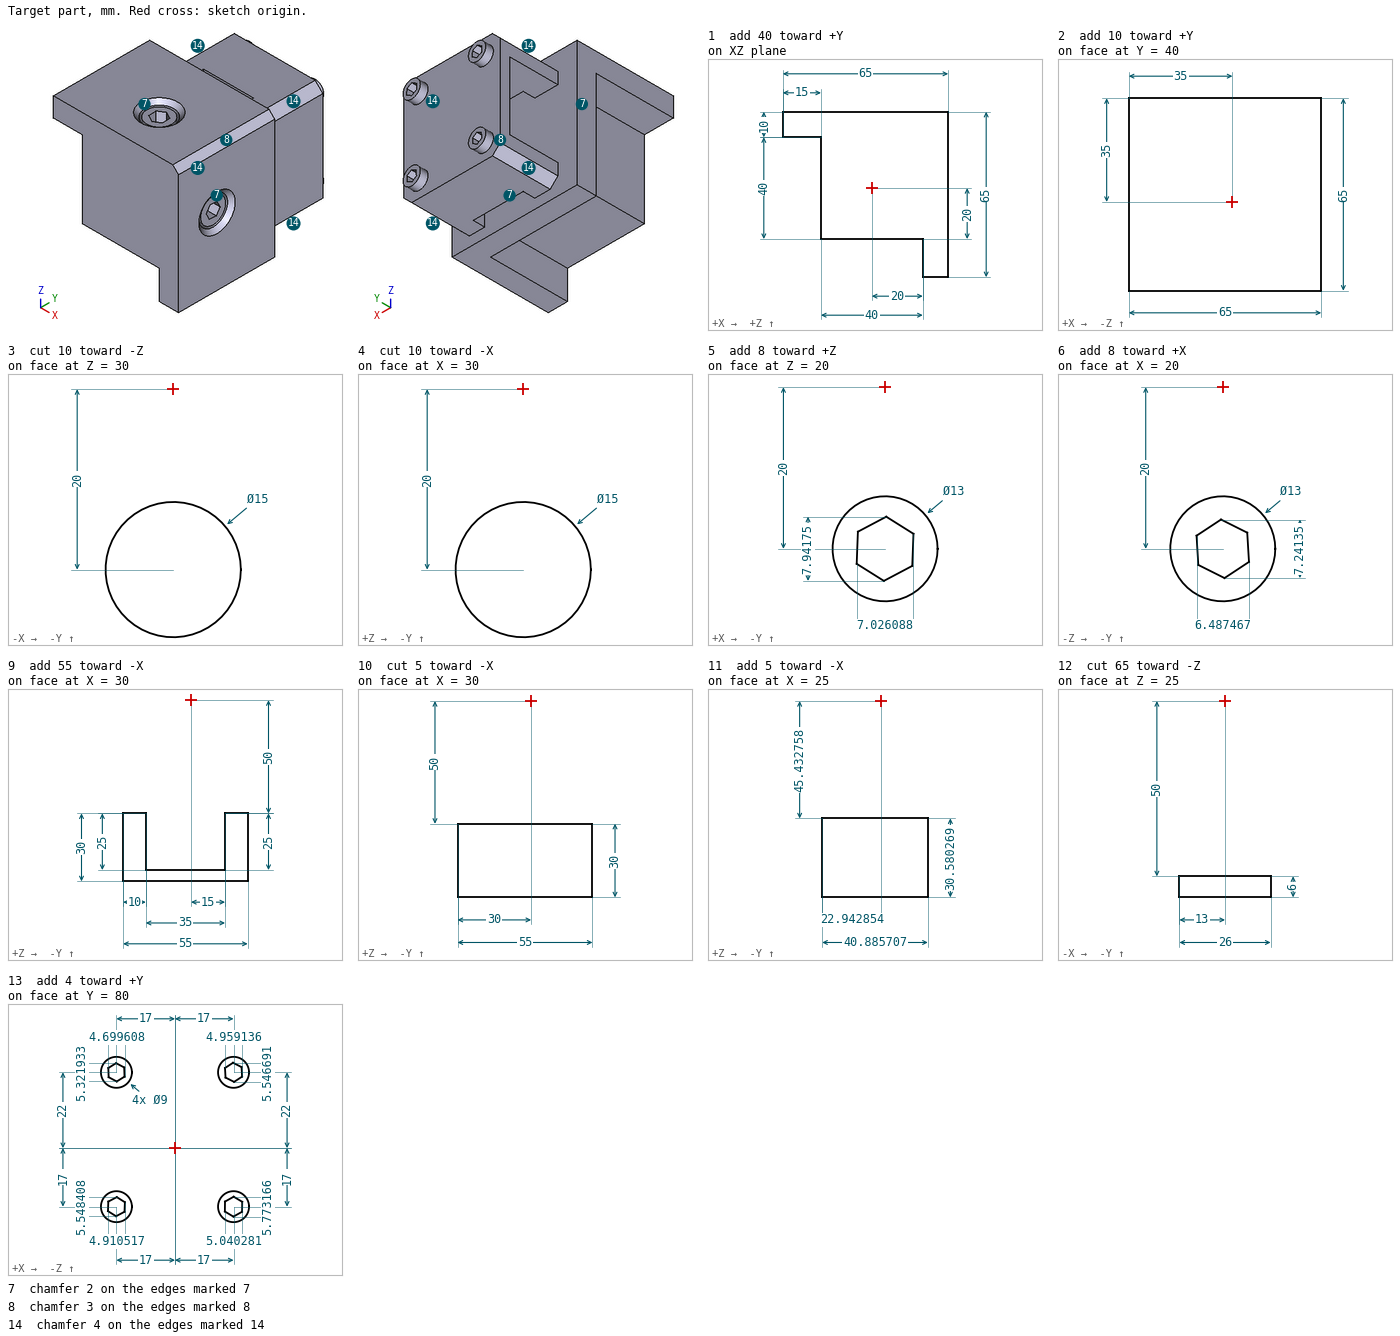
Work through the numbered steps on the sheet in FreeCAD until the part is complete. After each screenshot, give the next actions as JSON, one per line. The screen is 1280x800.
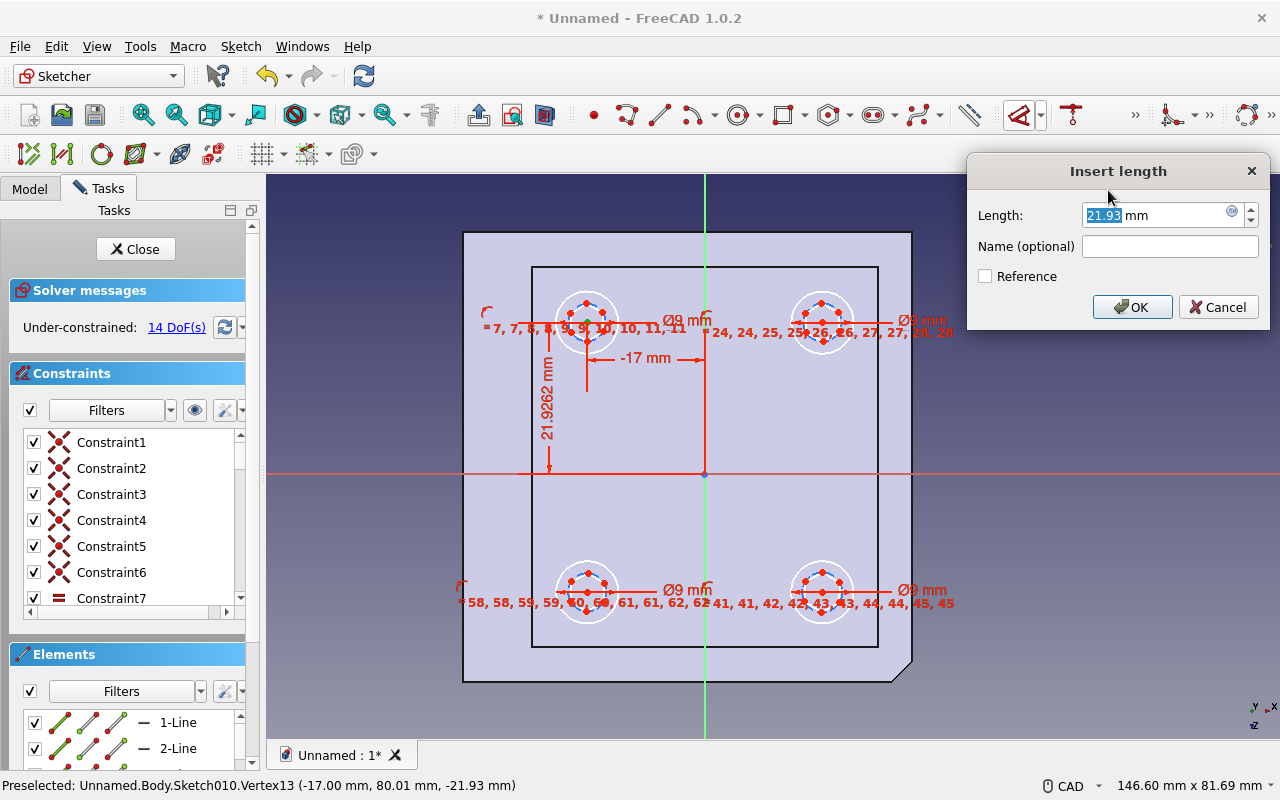
{"action": "type", "text": "22"}
{"action": "key", "text": "Return"}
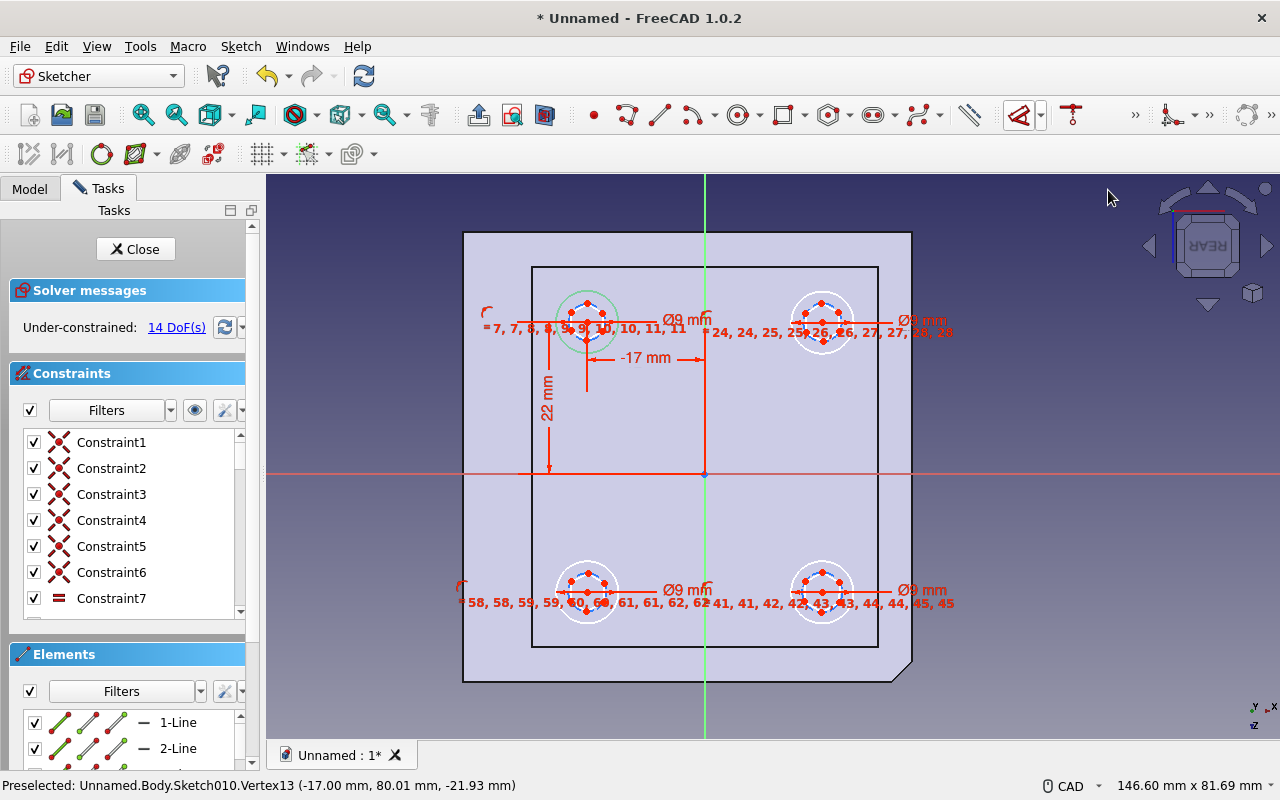
{"action": "left_click", "coordinate": [822, 323]}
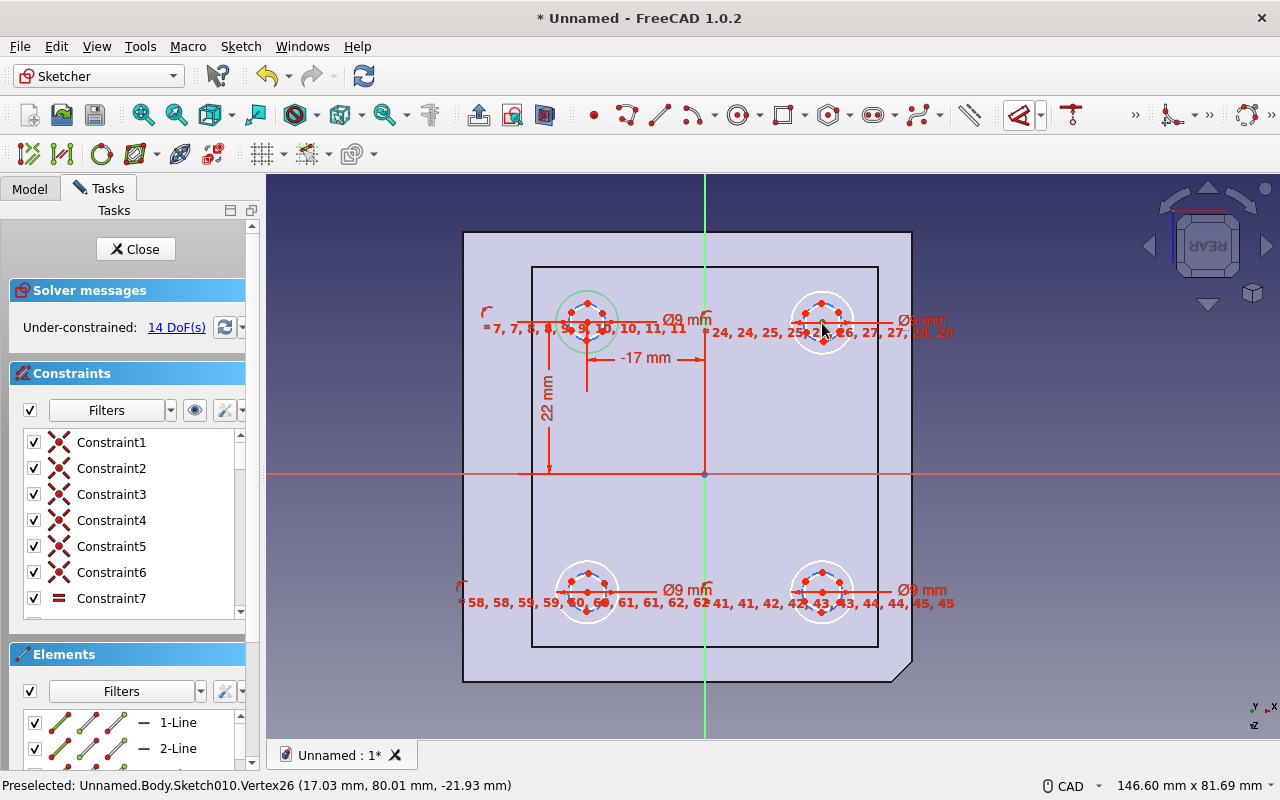
{"action": "left_click", "coordinate": [1040, 116]}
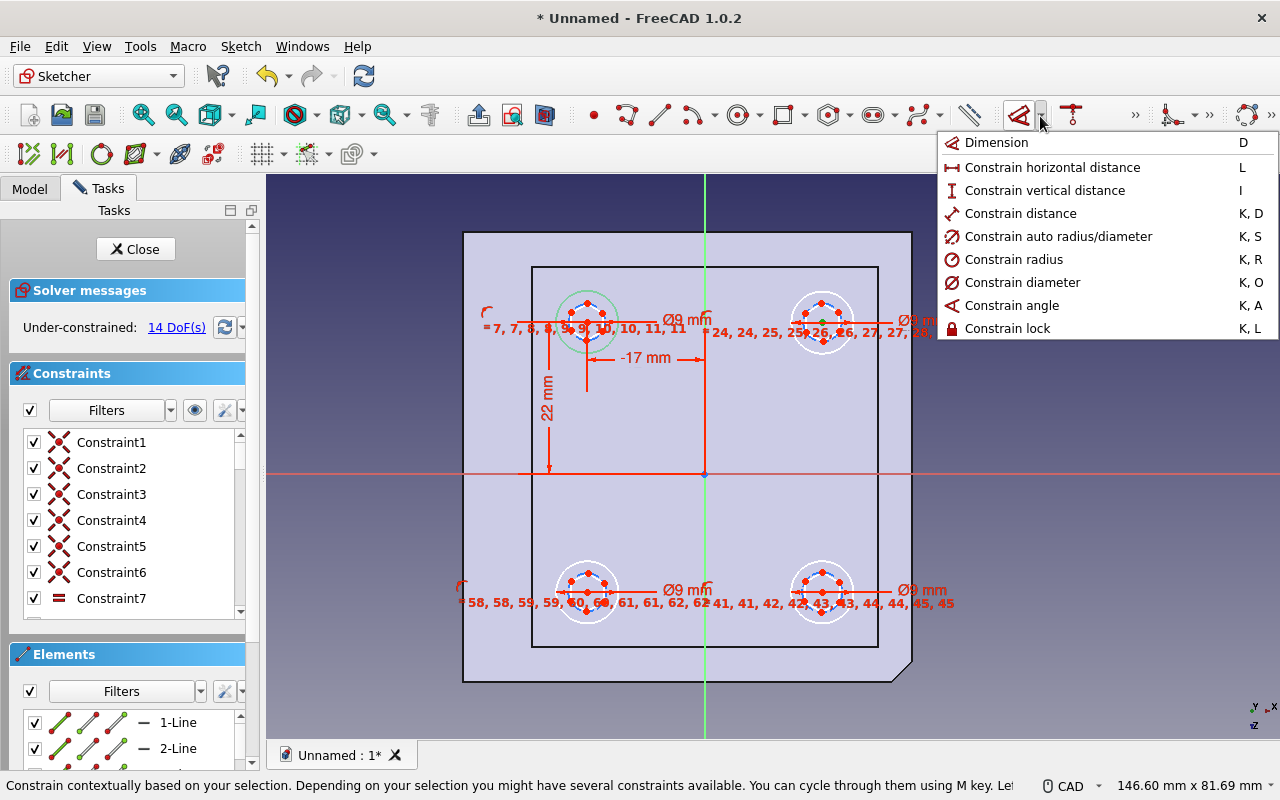
{"action": "left_click", "coordinate": [1108, 168]}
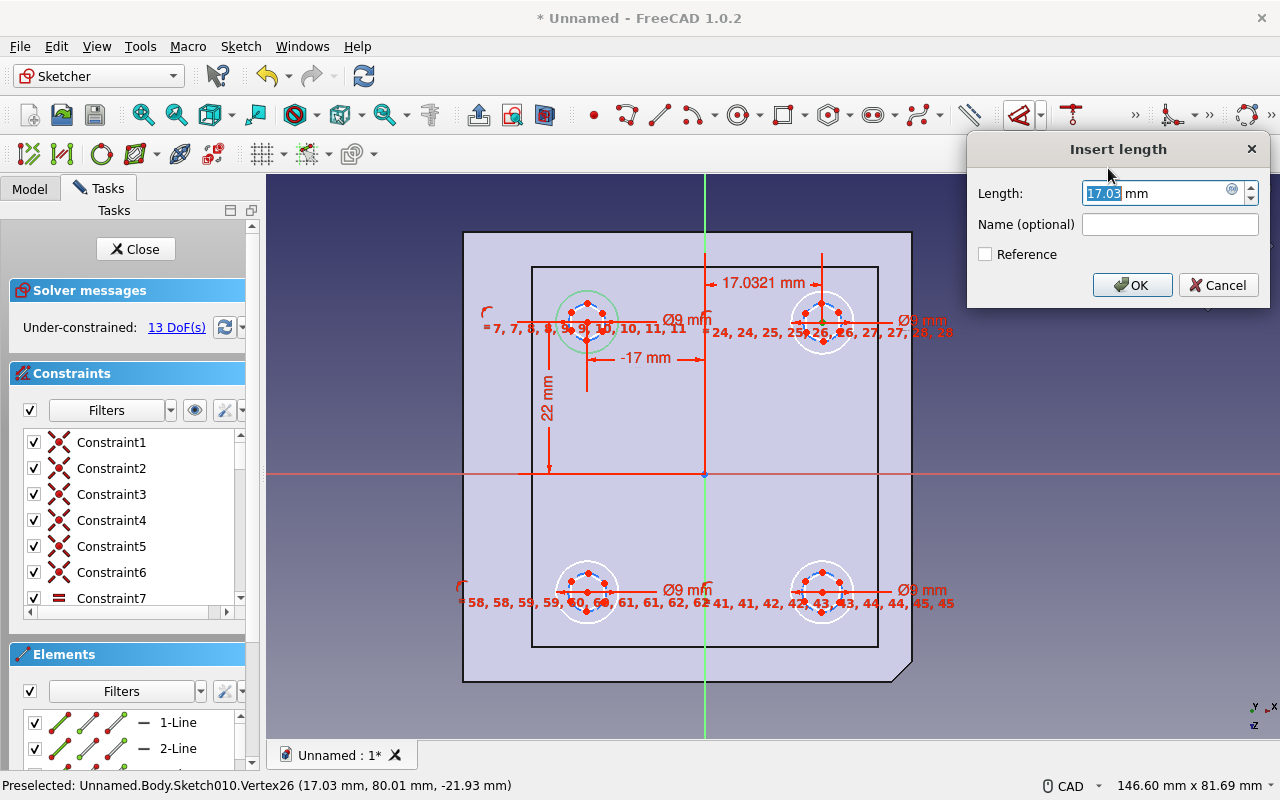
{"action": "type", "text": "17"}
{"action": "key", "text": "Return"}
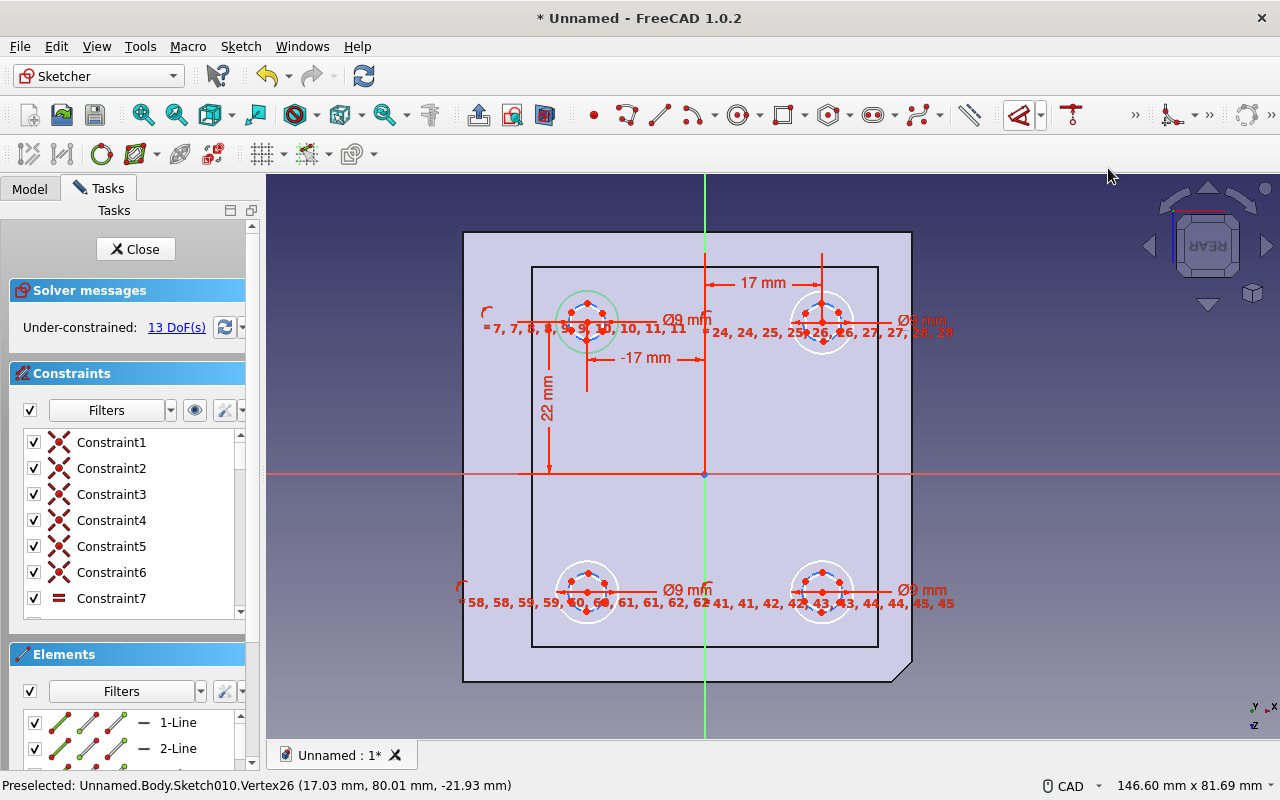
{"action": "left_click", "coordinate": [822, 323]}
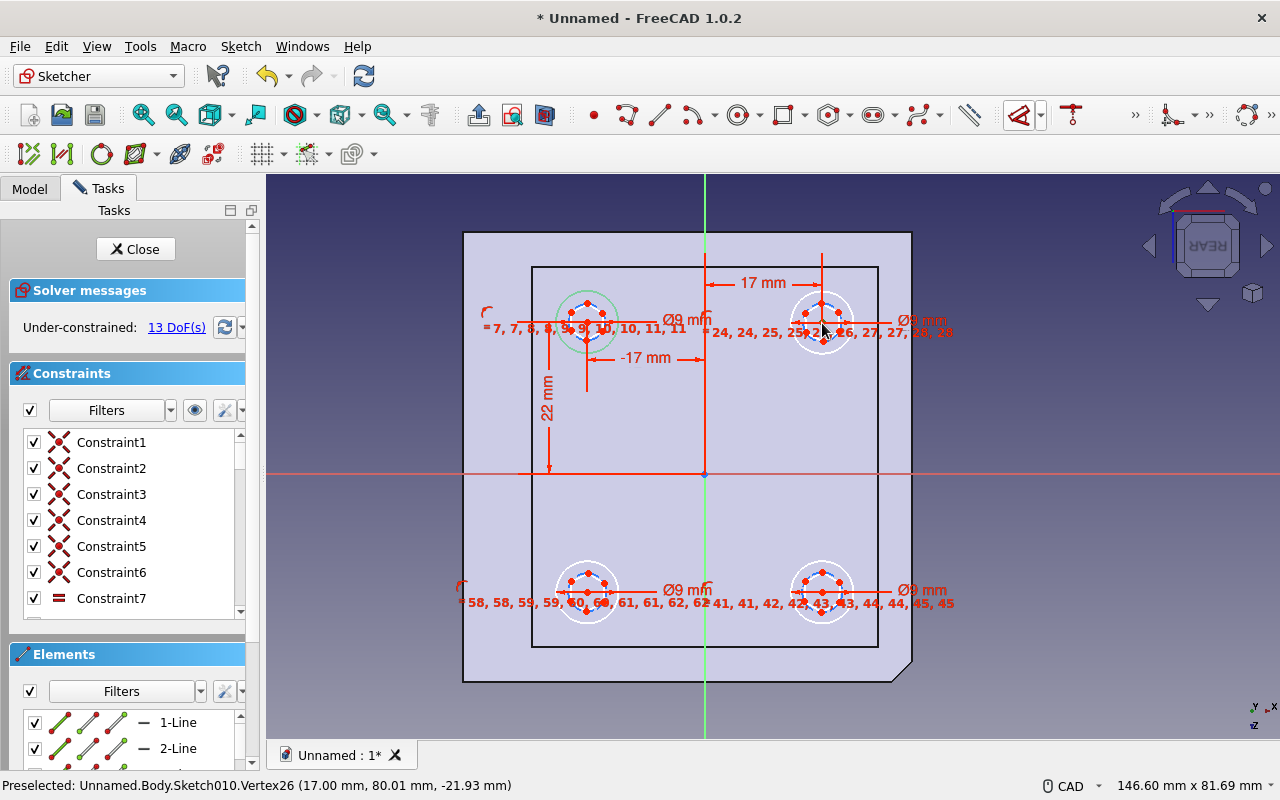
{"action": "left_click", "coordinate": [1040, 116]}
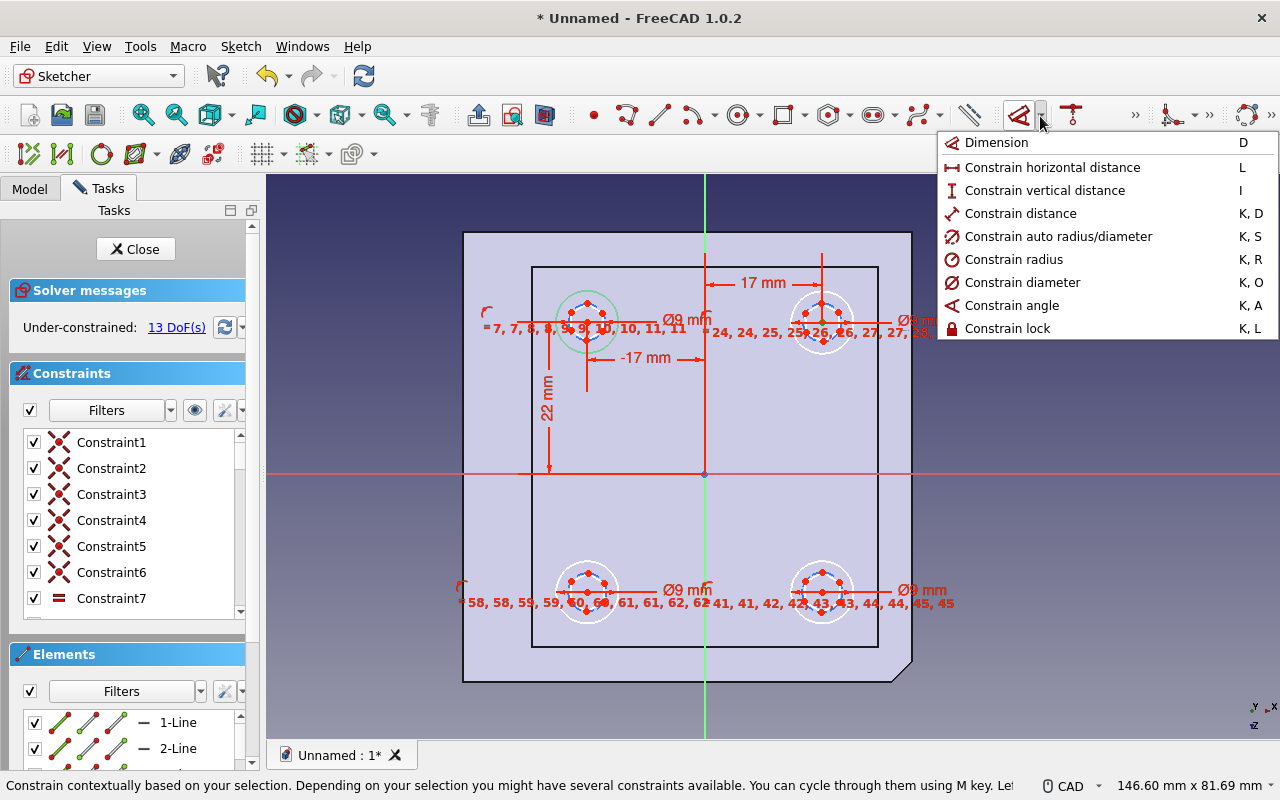
{"action": "left_click", "coordinate": [1108, 190]}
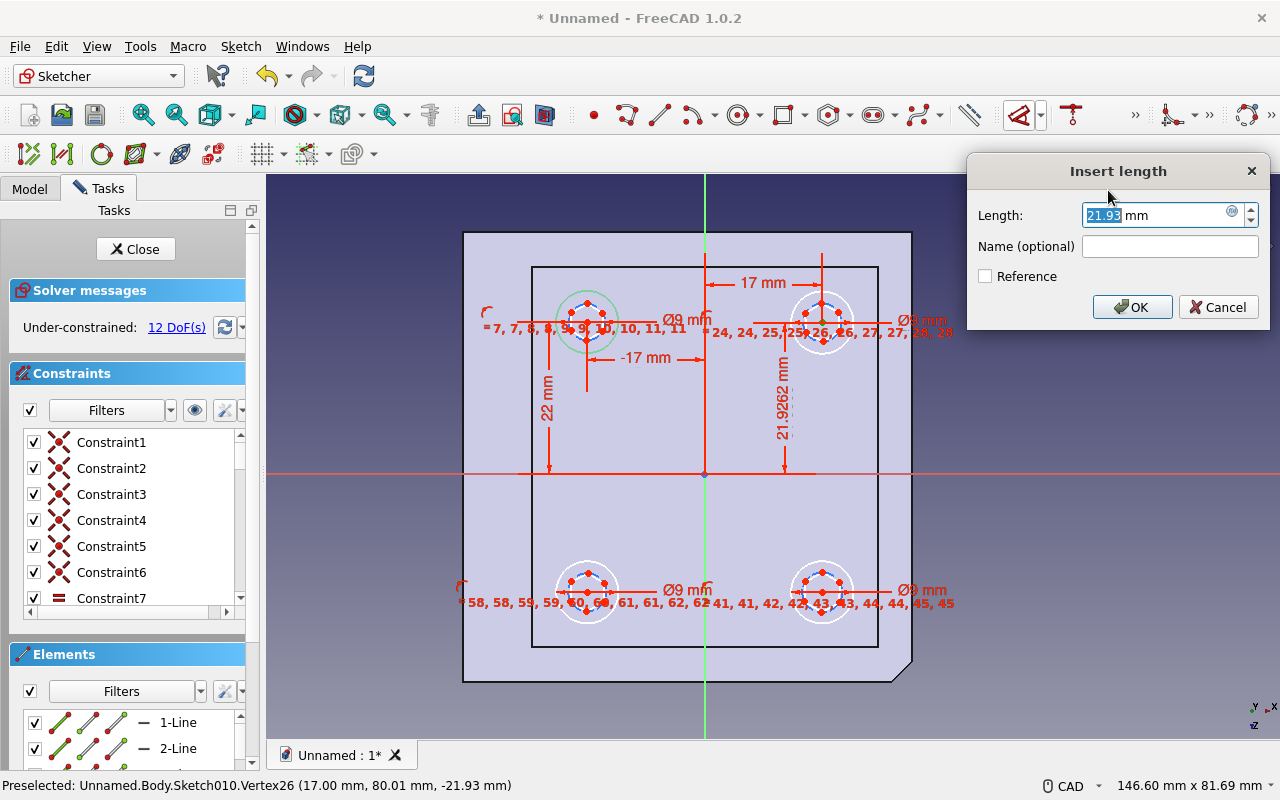
{"action": "type", "text": "22"}
{"action": "key", "text": "Return"}